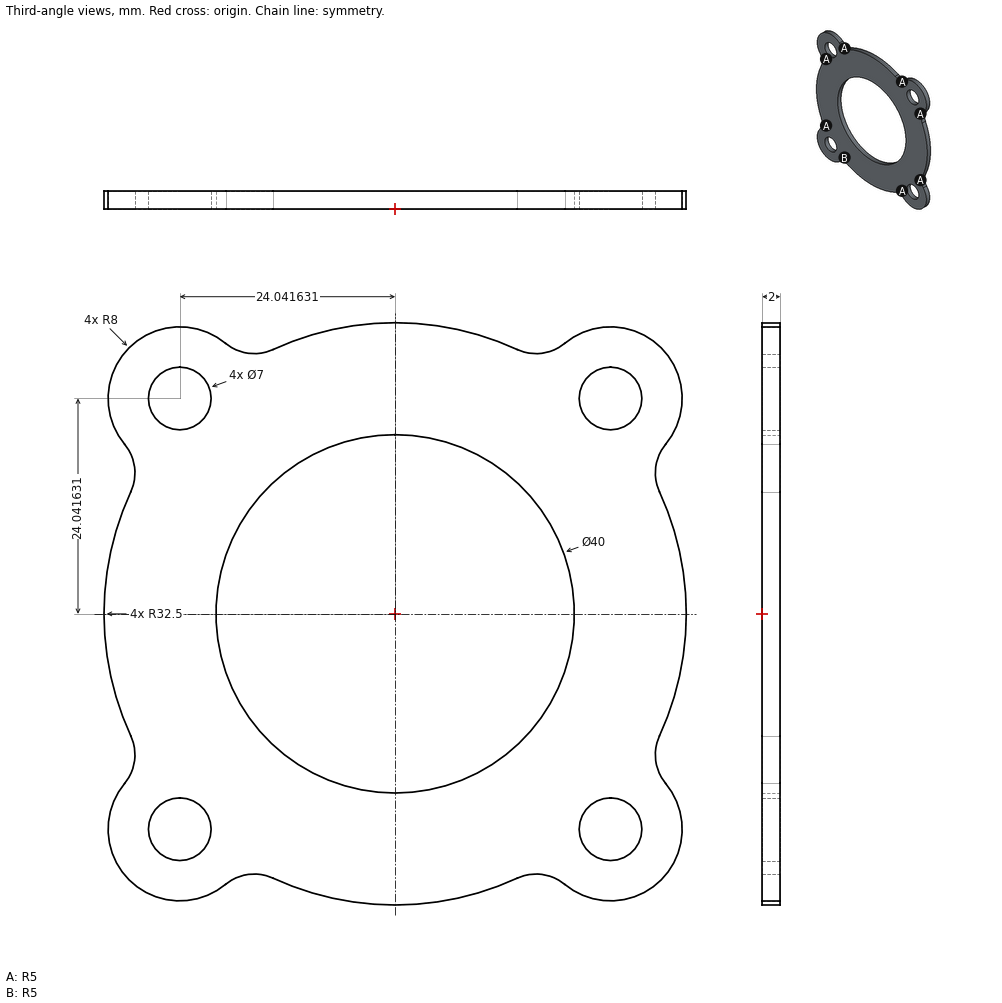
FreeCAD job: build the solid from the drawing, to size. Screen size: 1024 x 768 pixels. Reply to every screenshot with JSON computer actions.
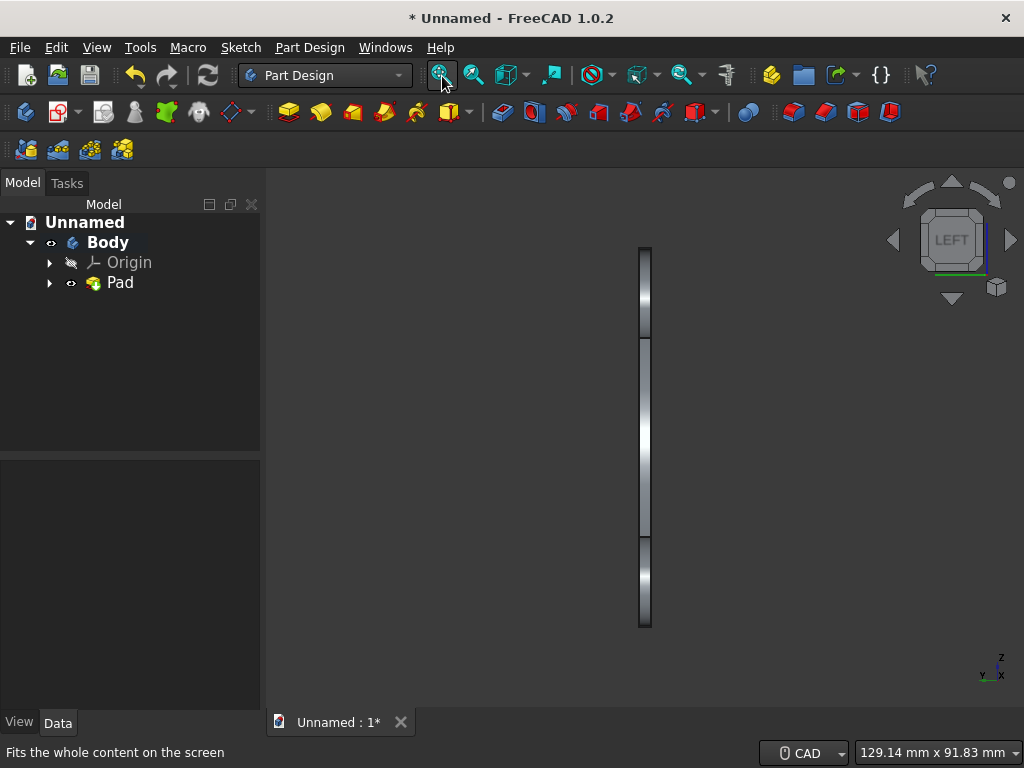
{"action": "key", "text": "v 3"}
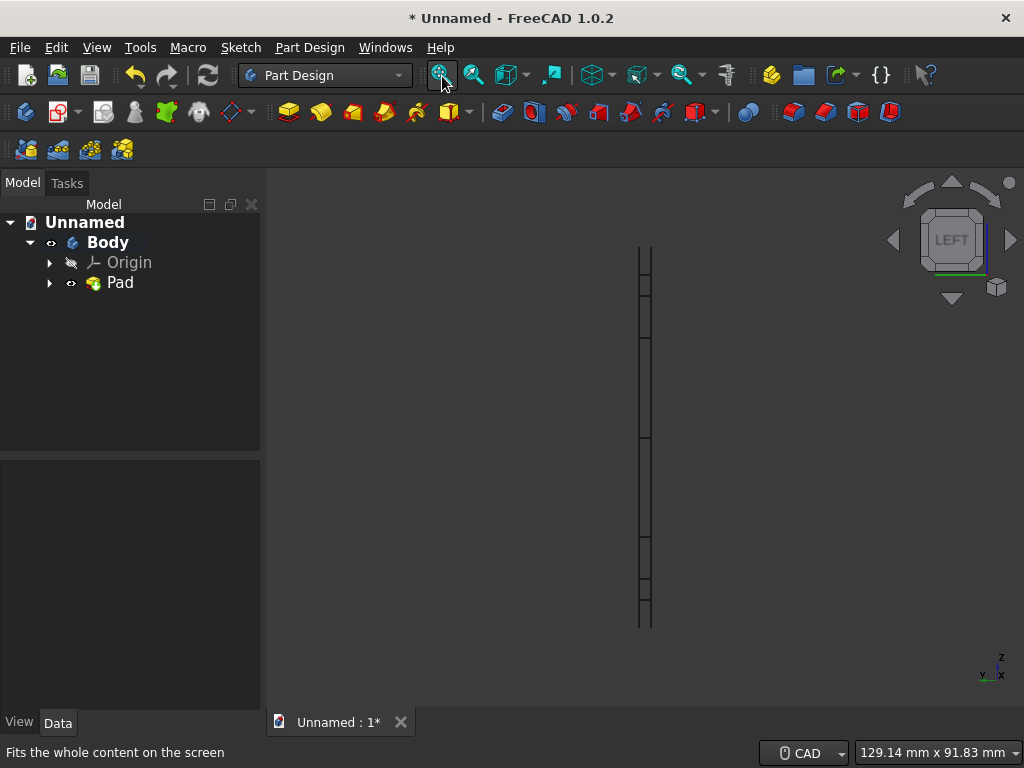
{"action": "key", "text": "0"}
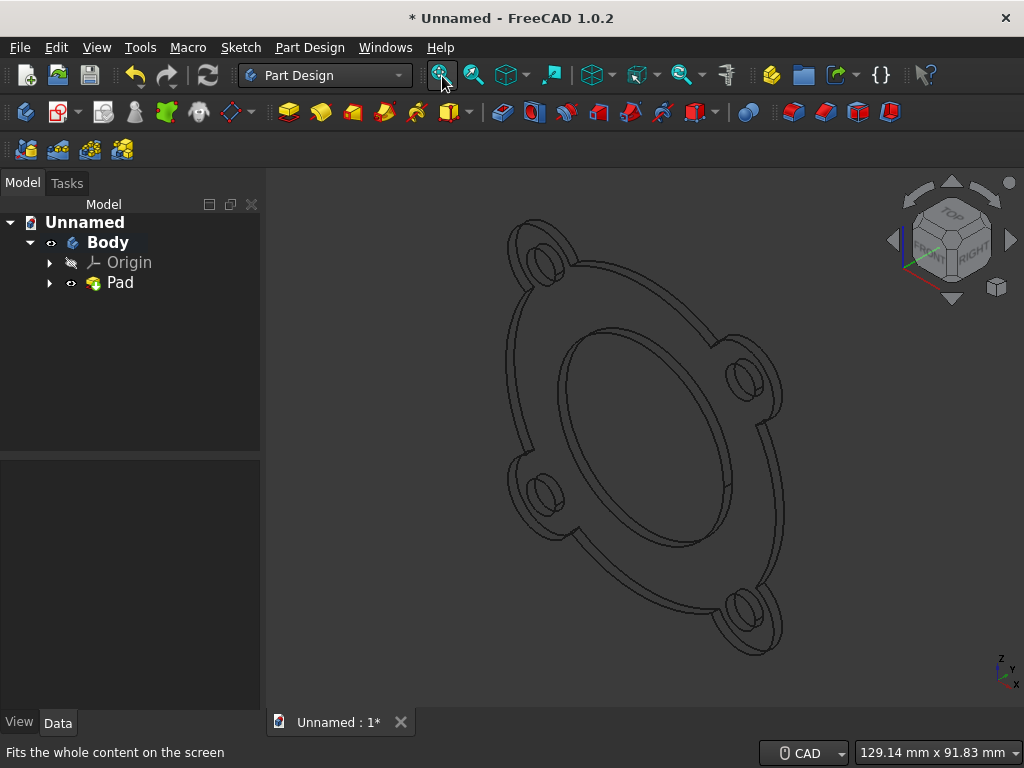
{"action": "left_click", "coordinate": [717, 609]}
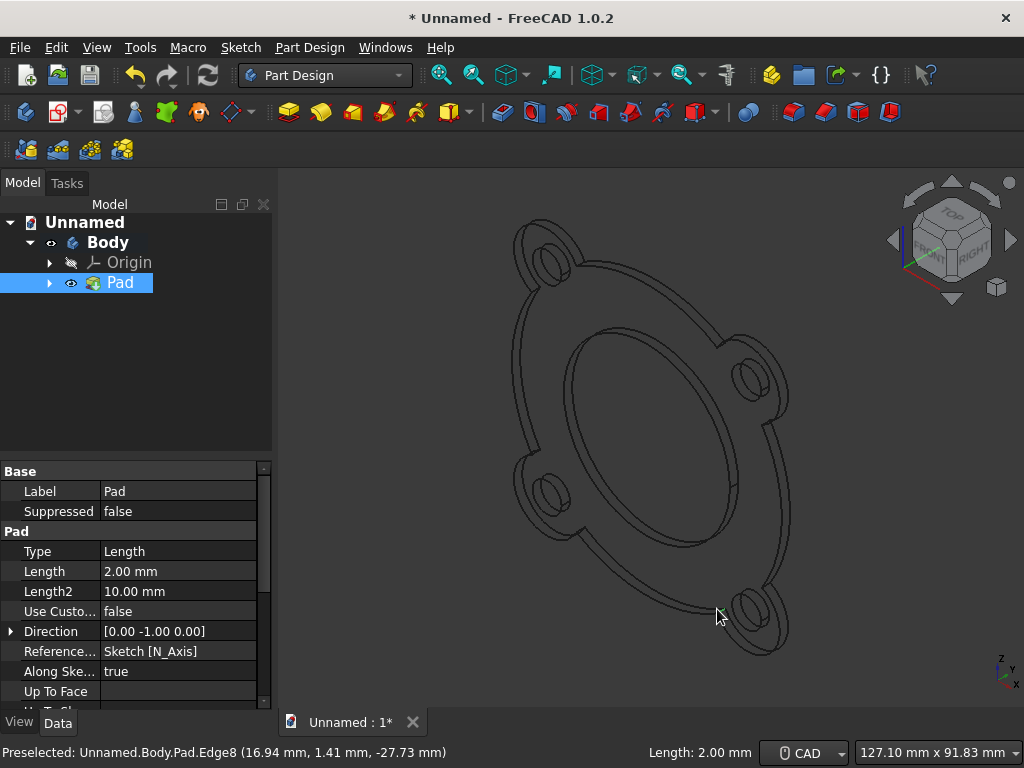
{"action": "left_click", "coordinate": [538, 288], "text": "ctrl"}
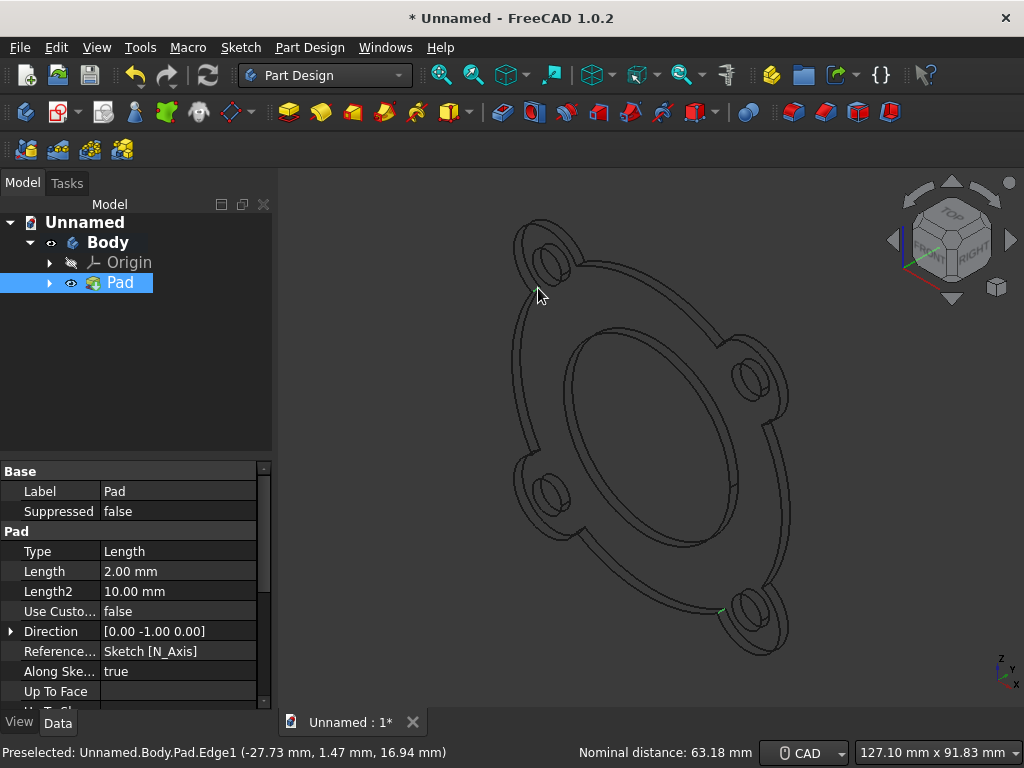
{"action": "left_click", "coordinate": [538, 450], "text": "ctrl"}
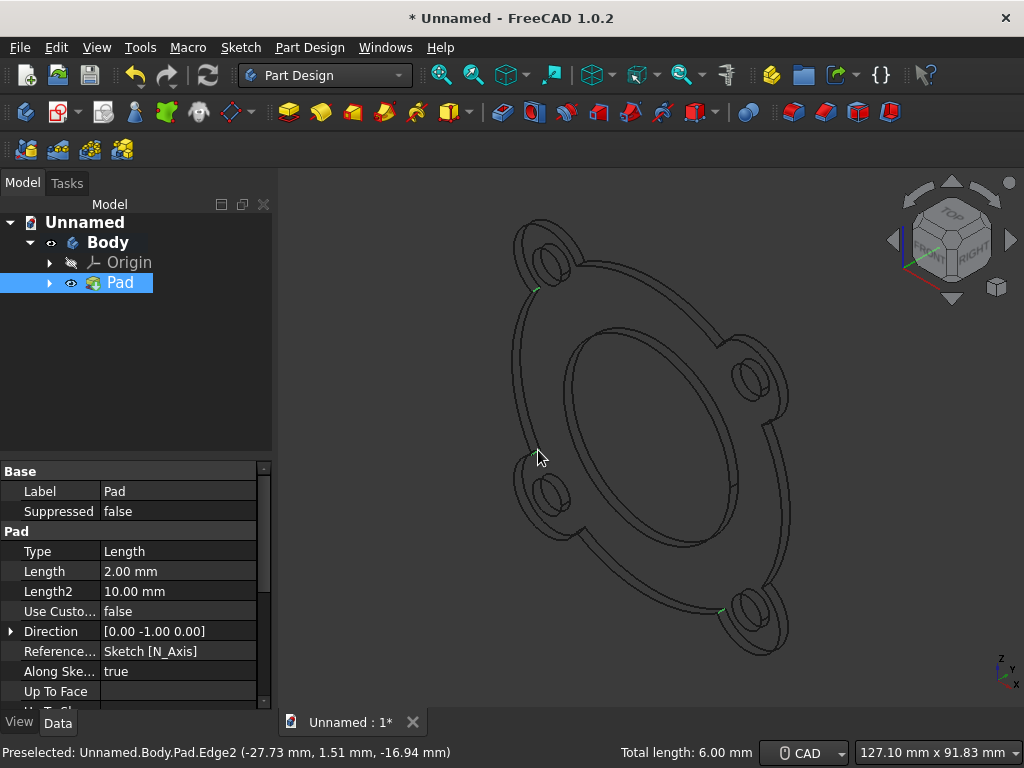
{"action": "scroll", "coordinate": [766, 584], "scroll_direction": "up", "scroll_amount": 7}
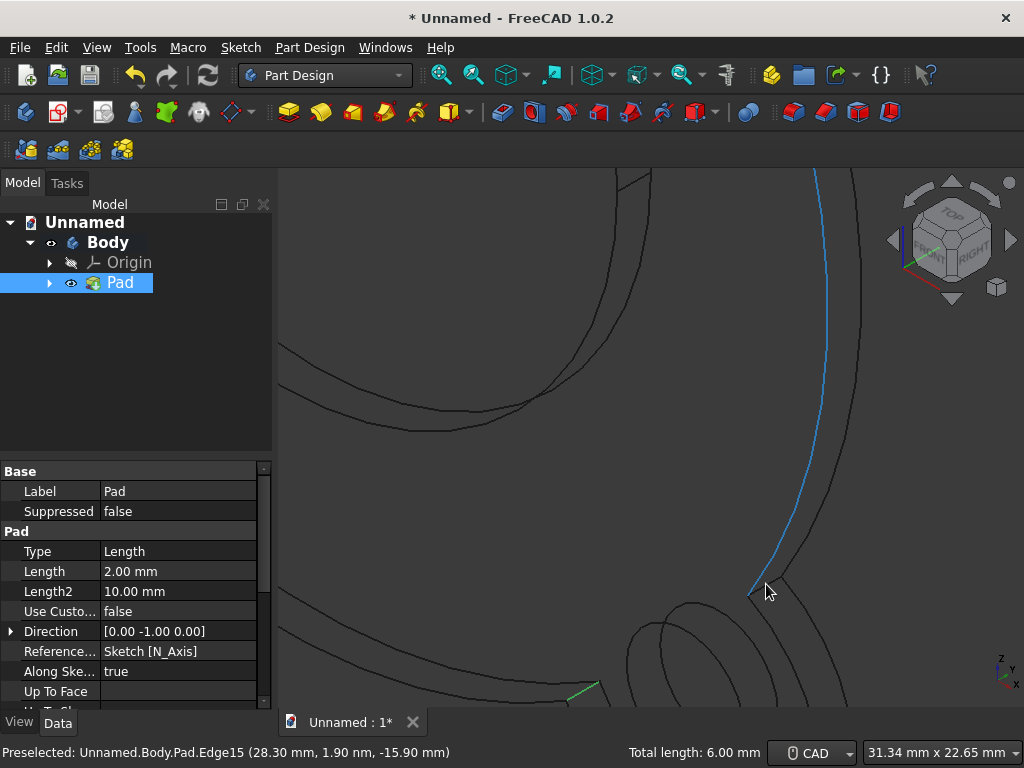
{"action": "left_click", "coordinate": [764, 585], "text": "ctrl"}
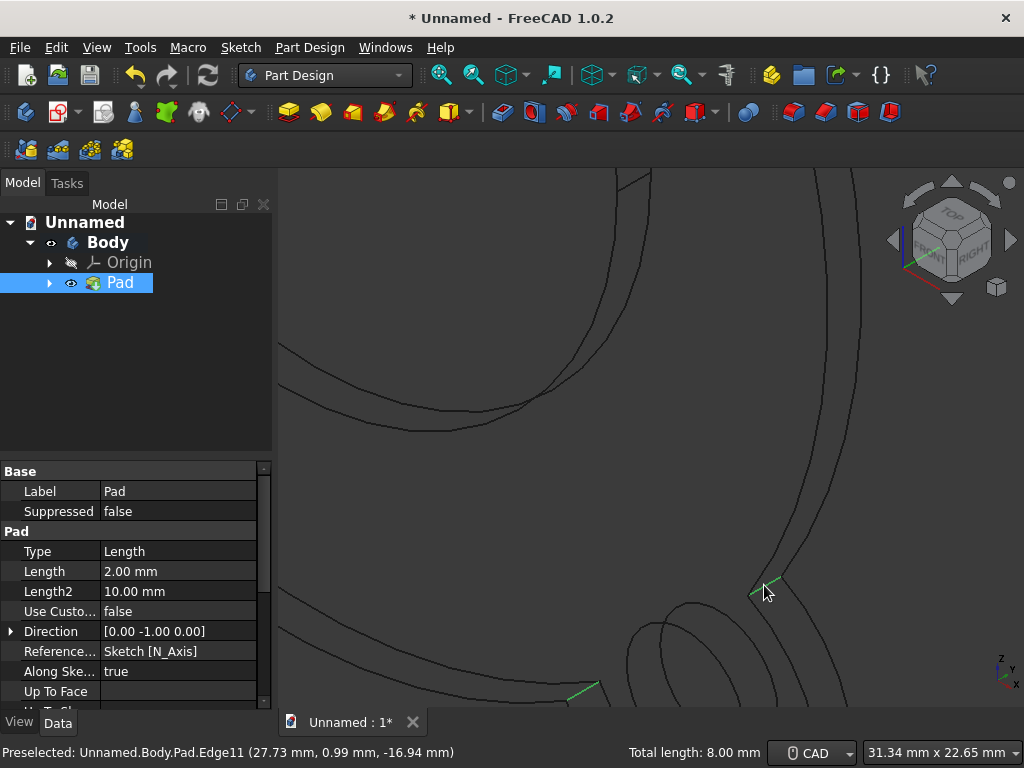
{"action": "left_click", "coordinate": [442, 76]}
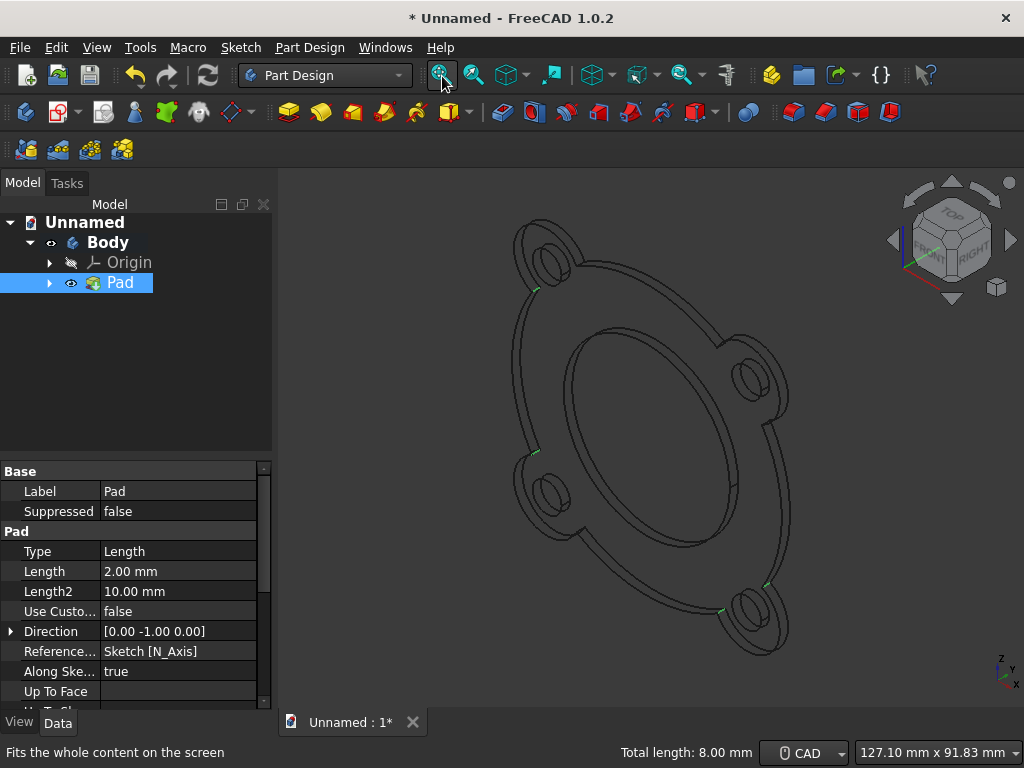
{"action": "key", "text": "2"}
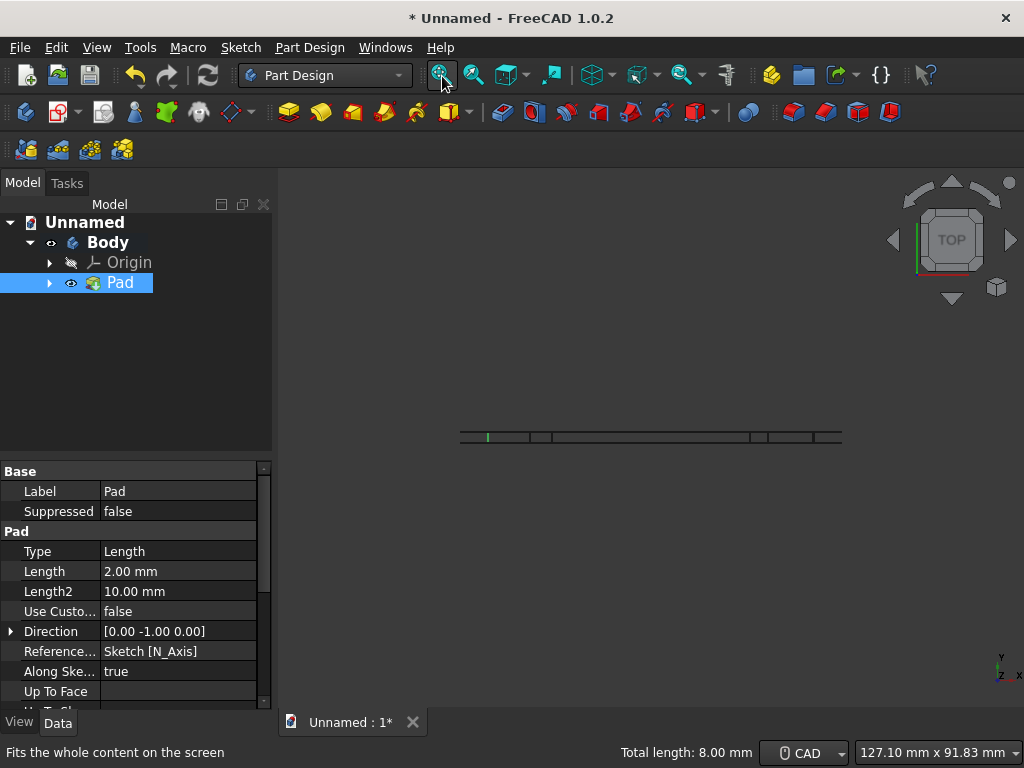
{"action": "scroll", "coordinate": [814, 436], "scroll_direction": "up", "scroll_amount": 7}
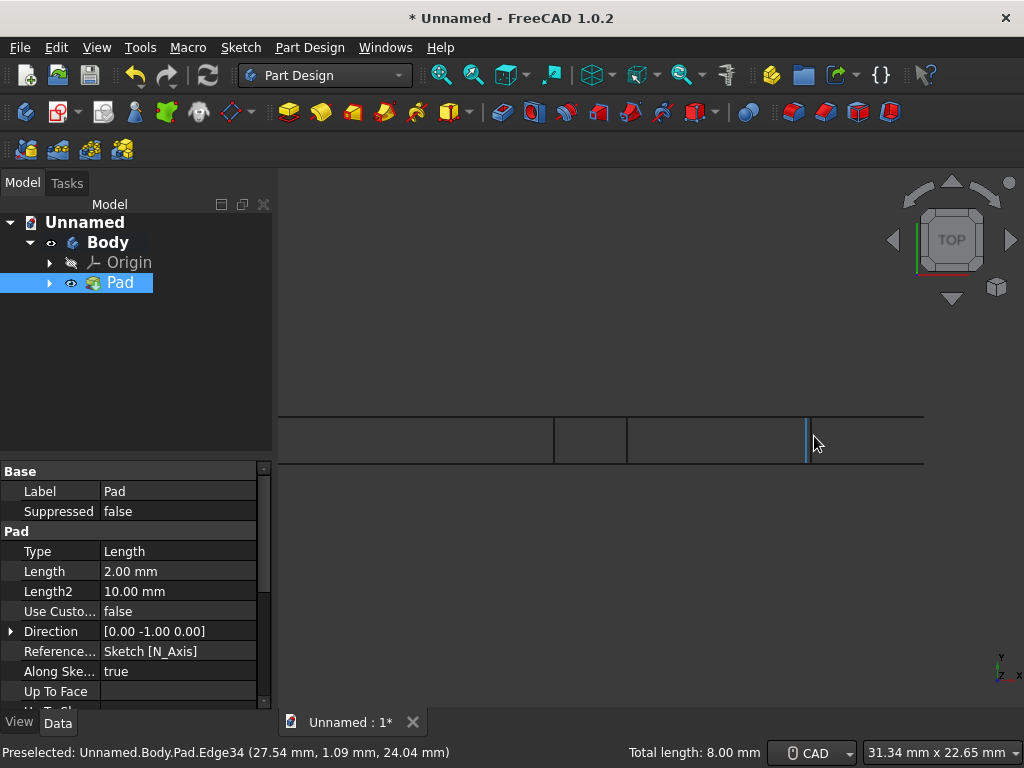
{"action": "left_click", "coordinate": [554, 440], "text": "ctrl"}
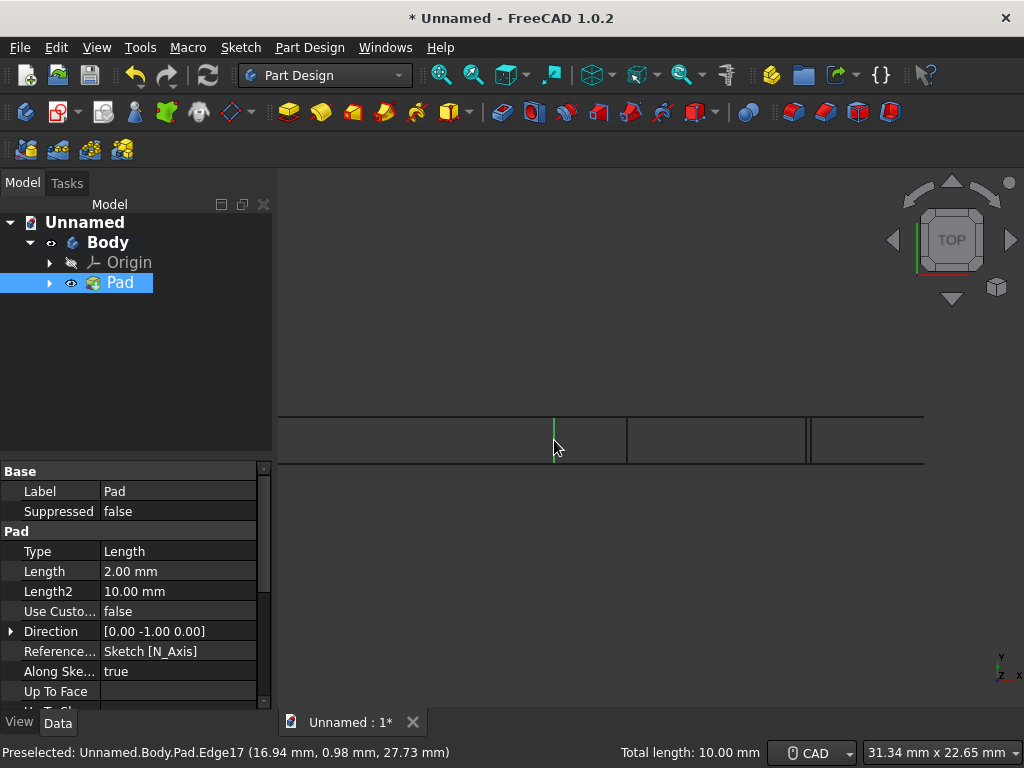
{"action": "left_click", "coordinate": [442, 76]}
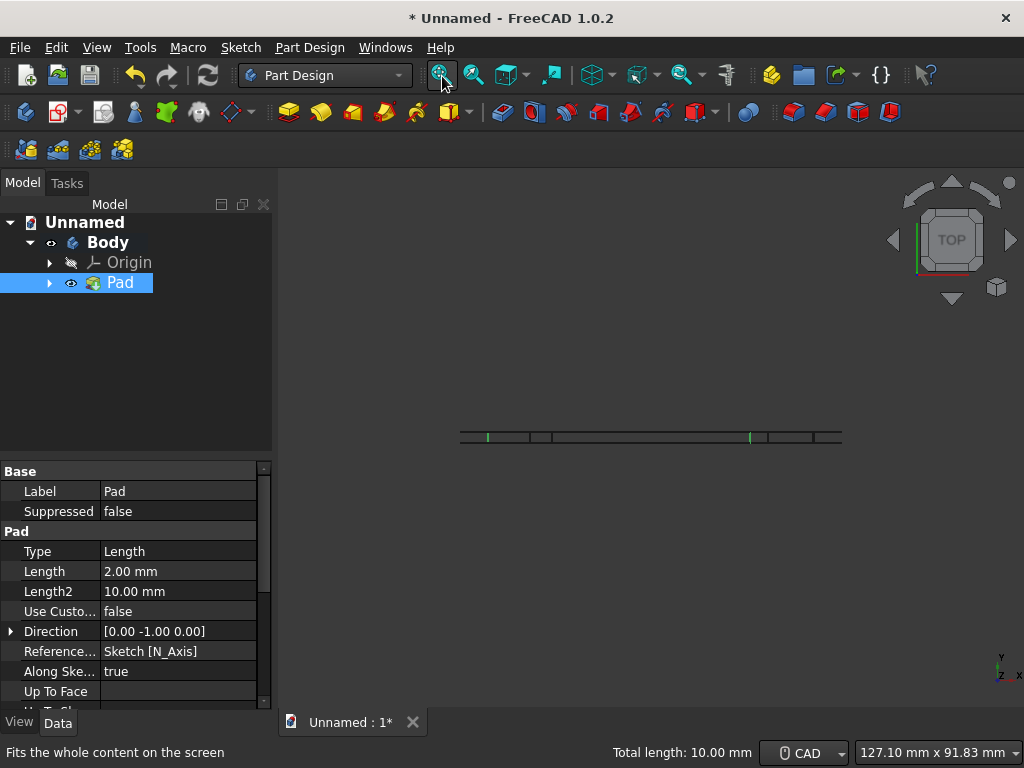
{"action": "key", "text": "1"}